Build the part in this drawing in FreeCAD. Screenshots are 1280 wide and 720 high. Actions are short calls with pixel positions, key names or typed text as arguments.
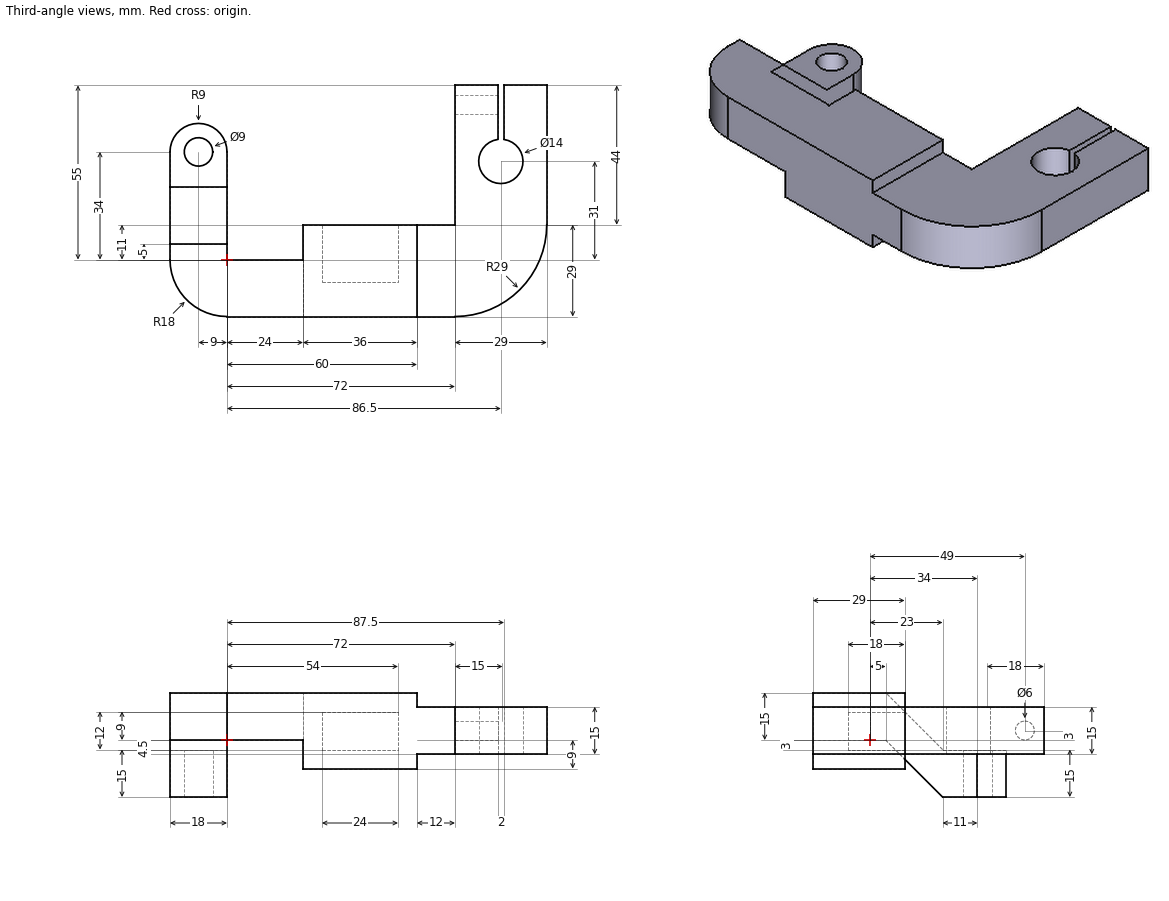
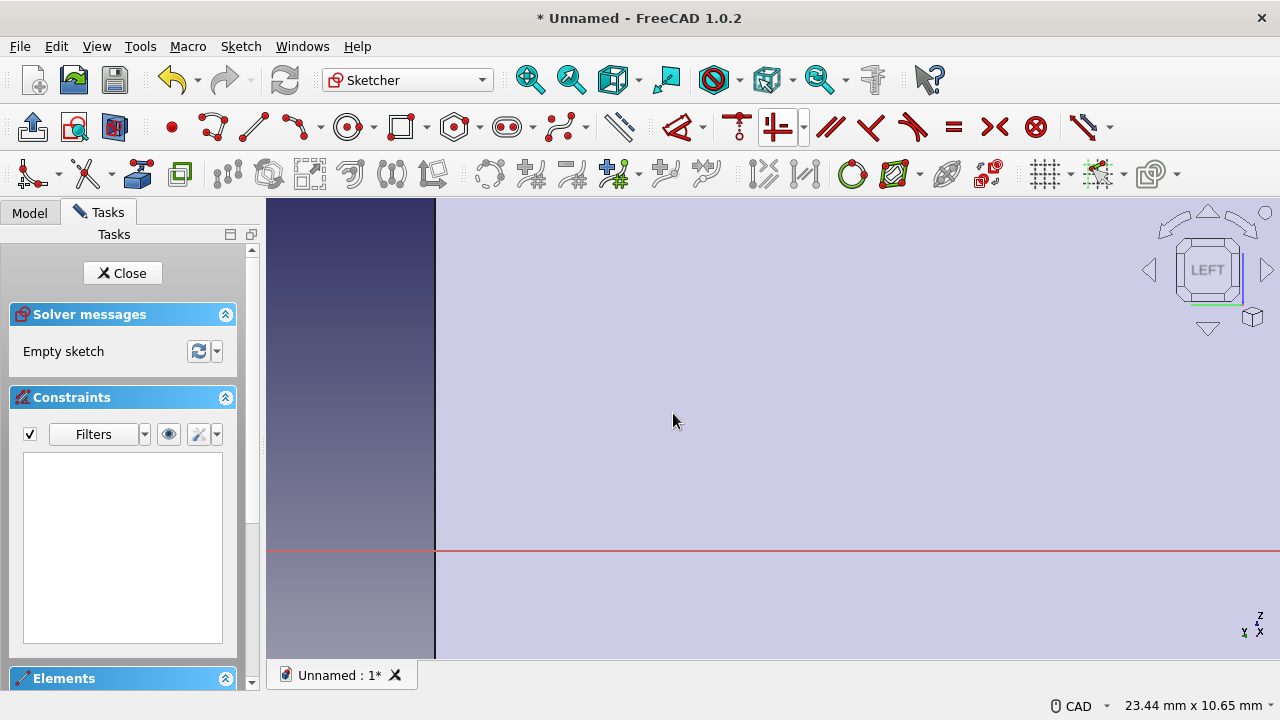
click(348, 128)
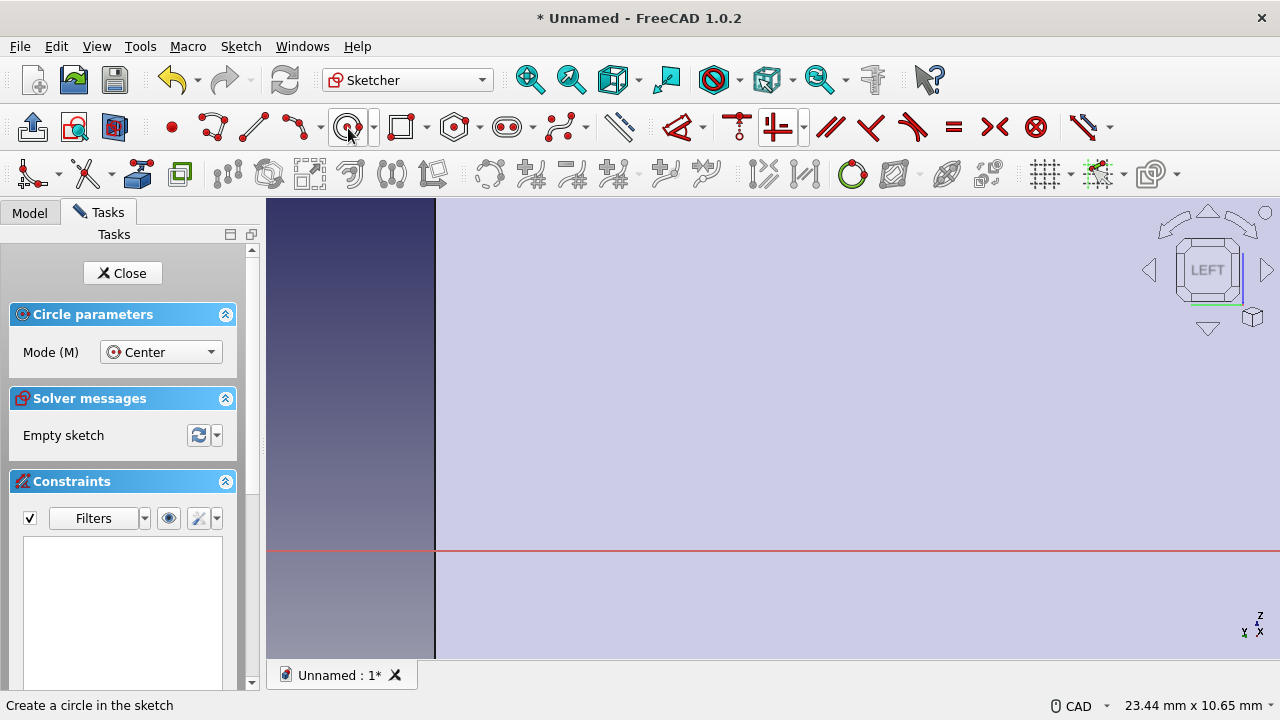
click(695, 421)
move(787, 329)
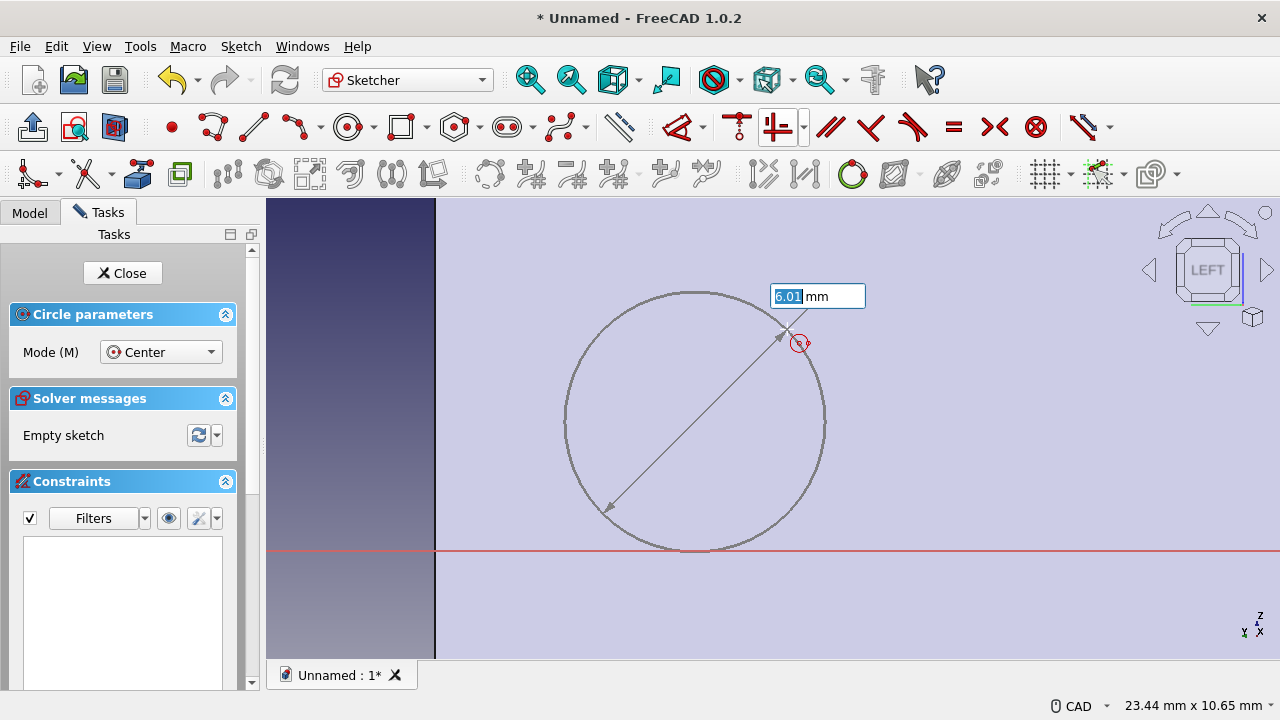
text(6)
key(Return)
key(Escape)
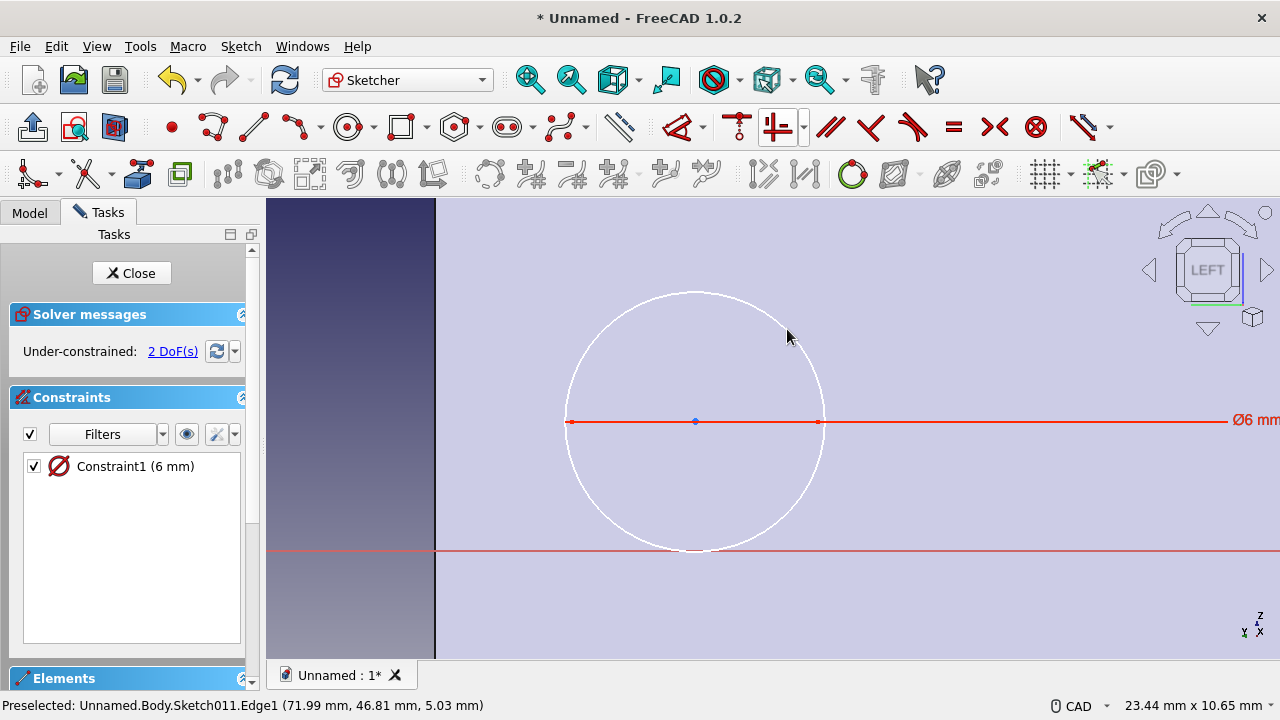
click(676, 128)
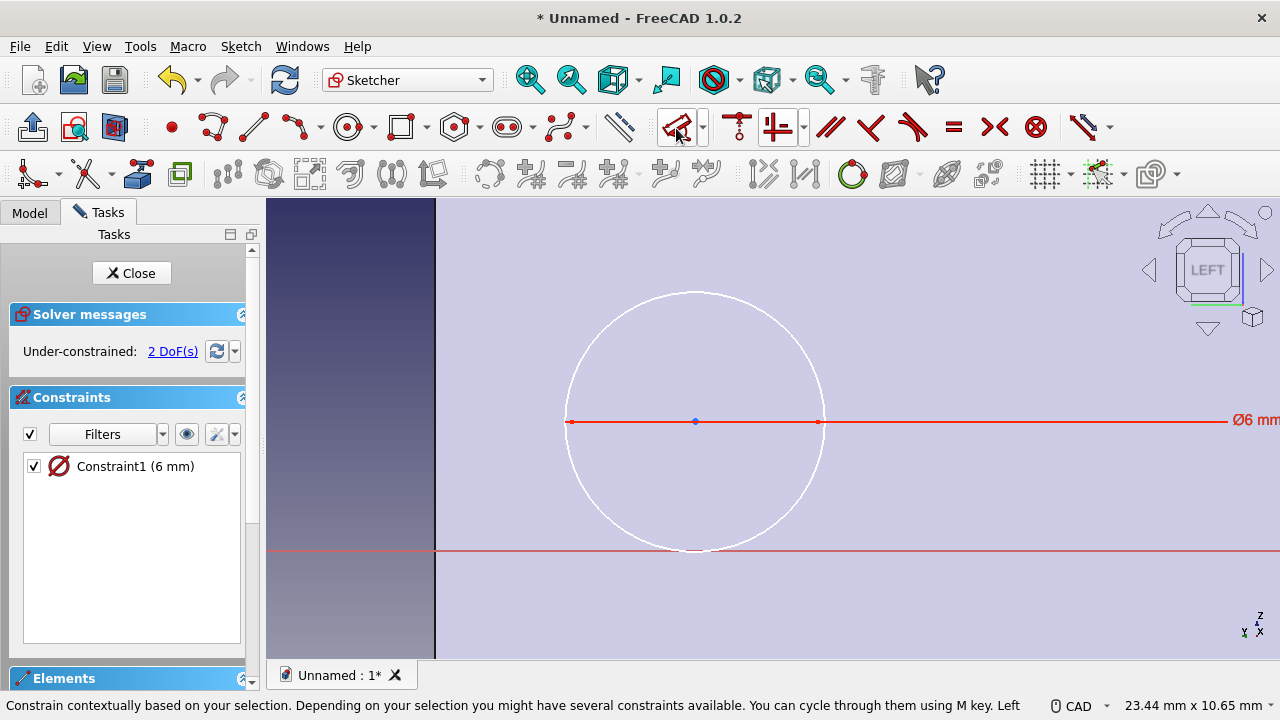
click(695, 422)
click(661, 486)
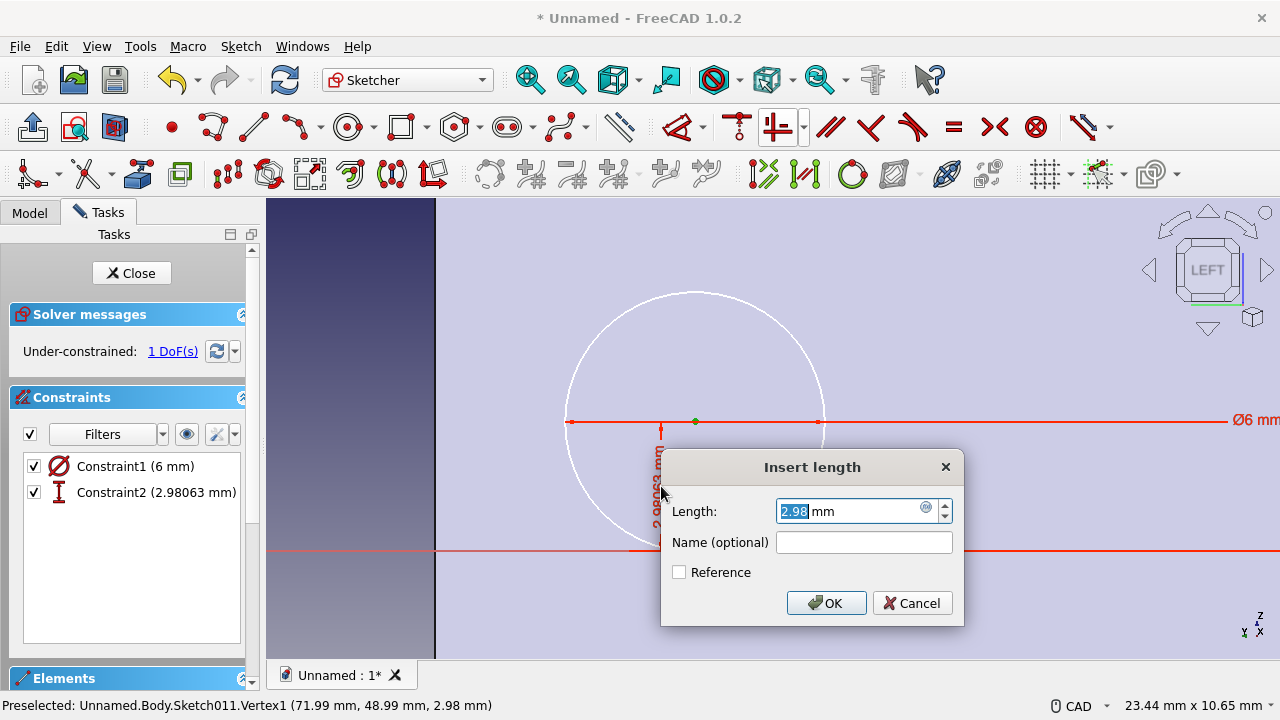
text(3)
key(Return)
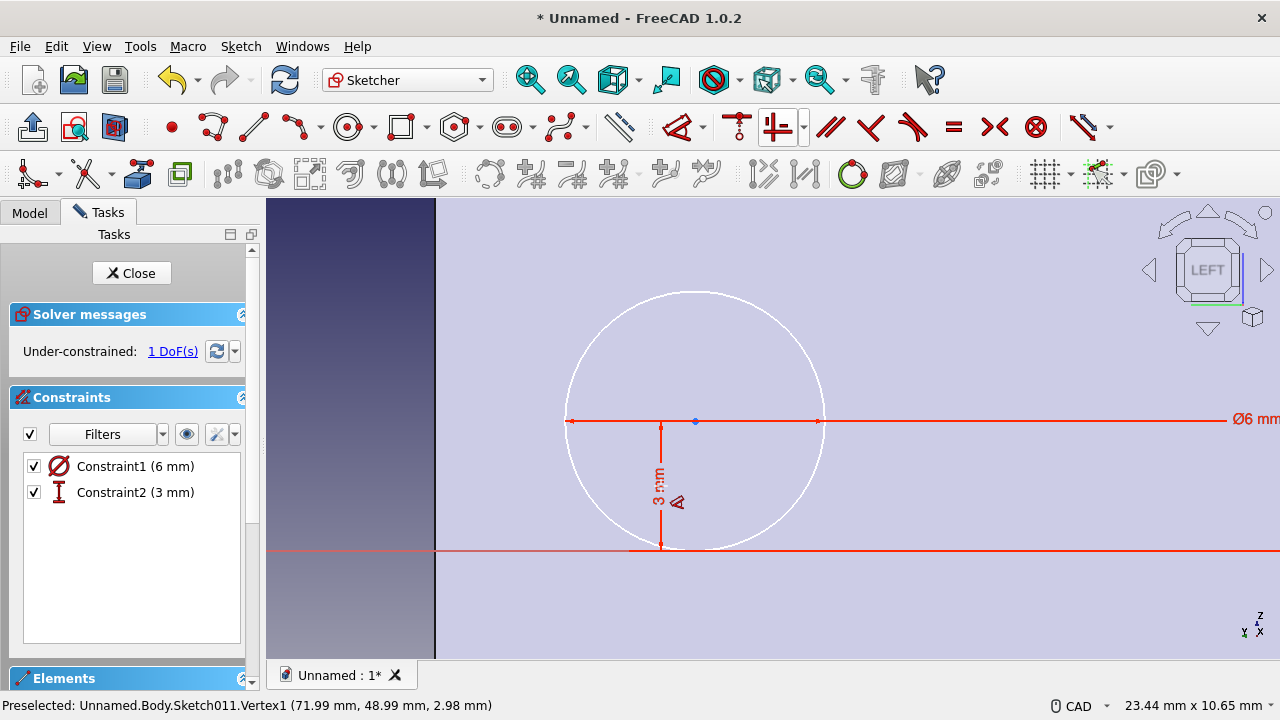
click(695, 421)
click(905, 585)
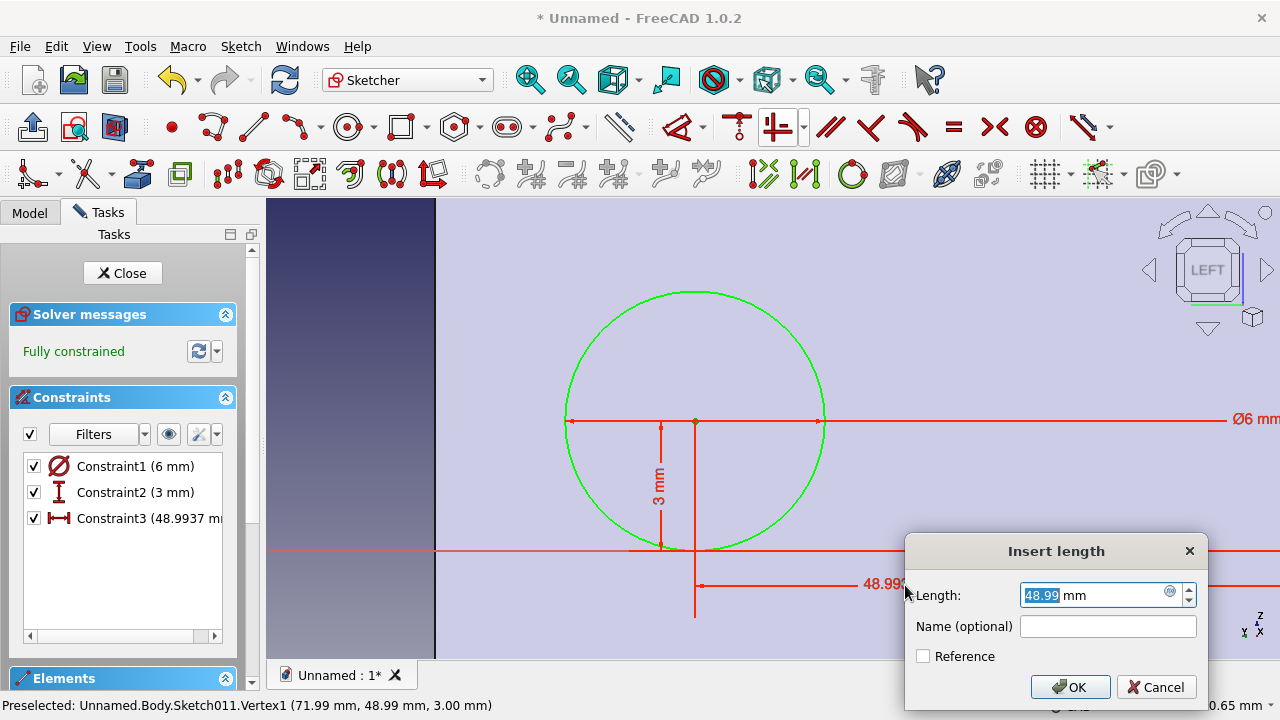
text(49)
key(Return)
key(Escape)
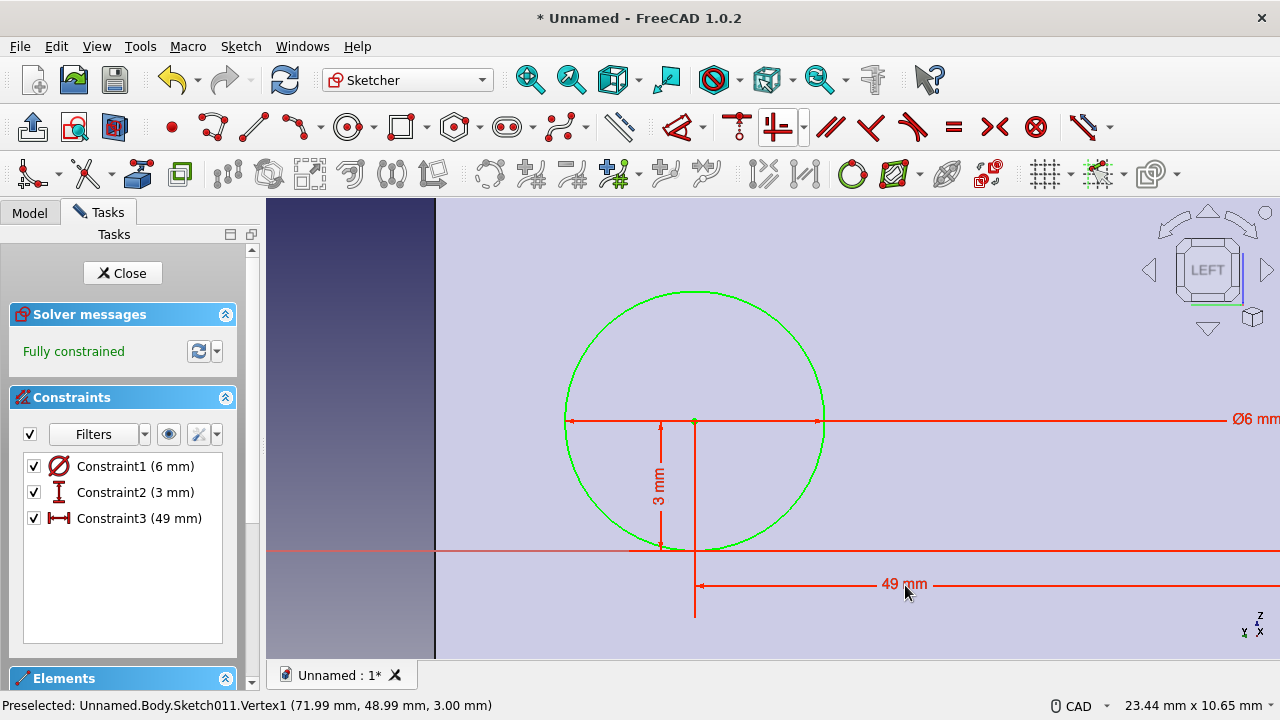
click(123, 273)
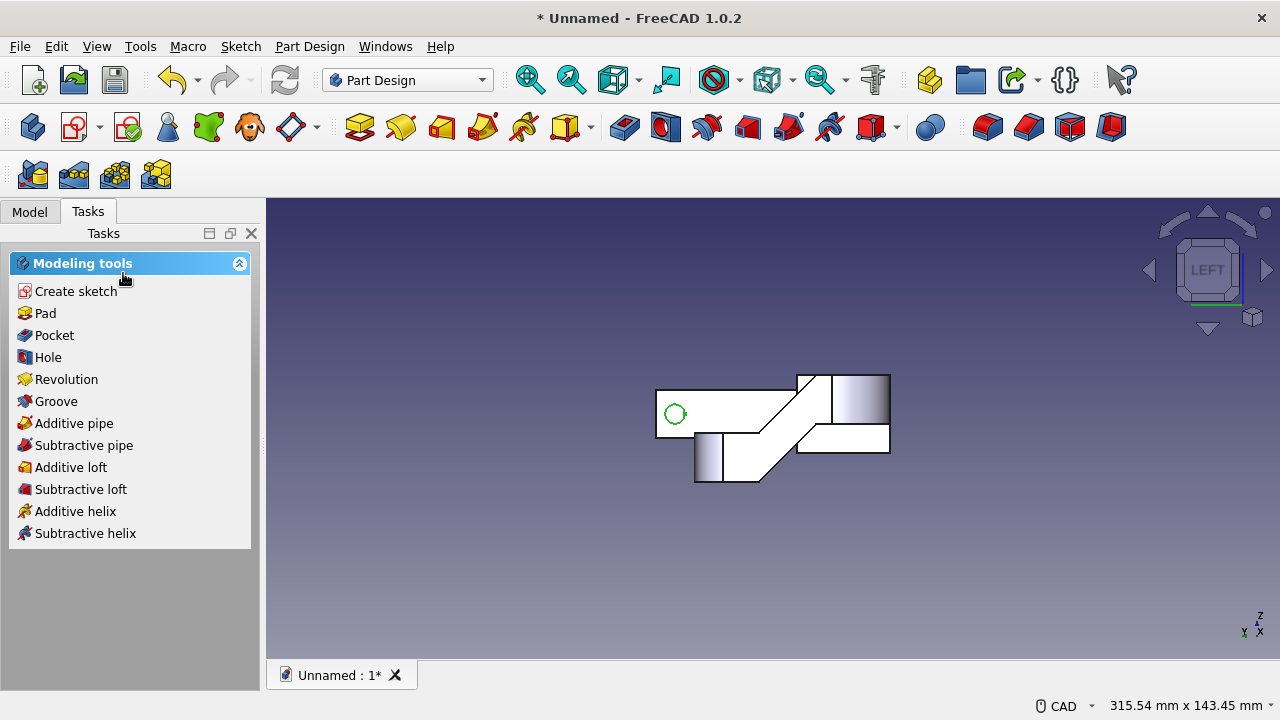
click(625, 128)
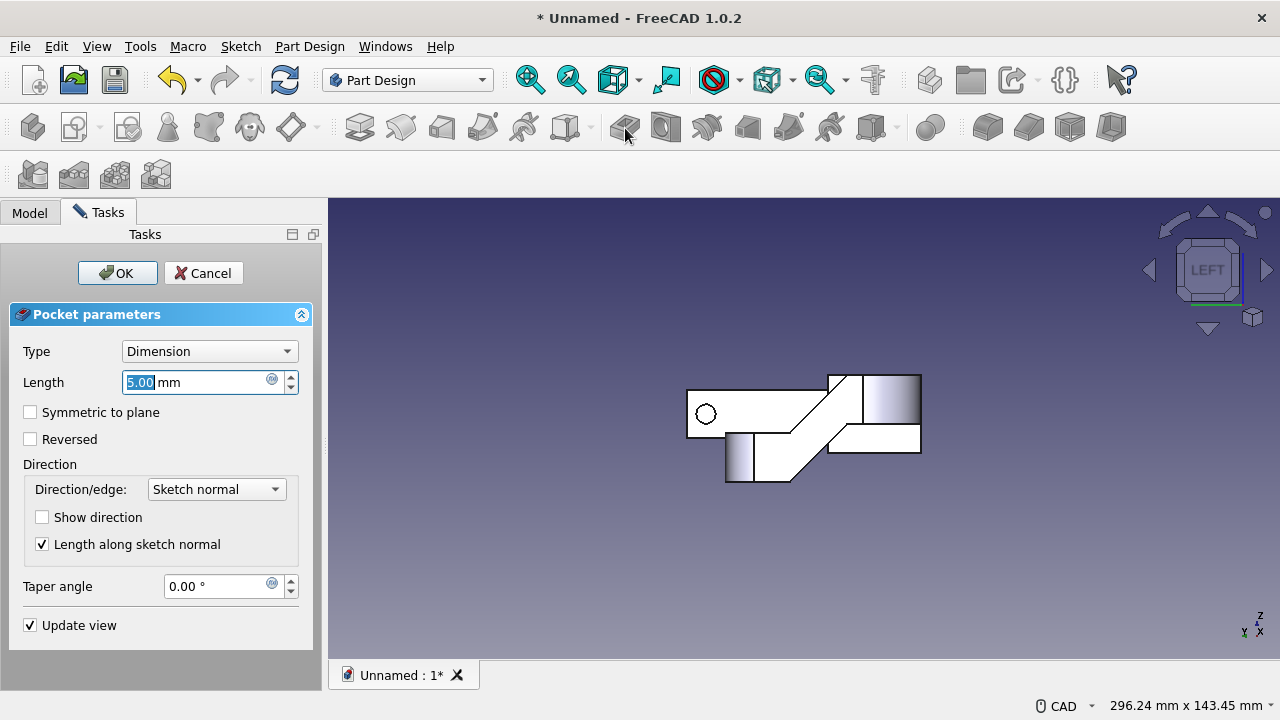
text(15)
key(Tab)